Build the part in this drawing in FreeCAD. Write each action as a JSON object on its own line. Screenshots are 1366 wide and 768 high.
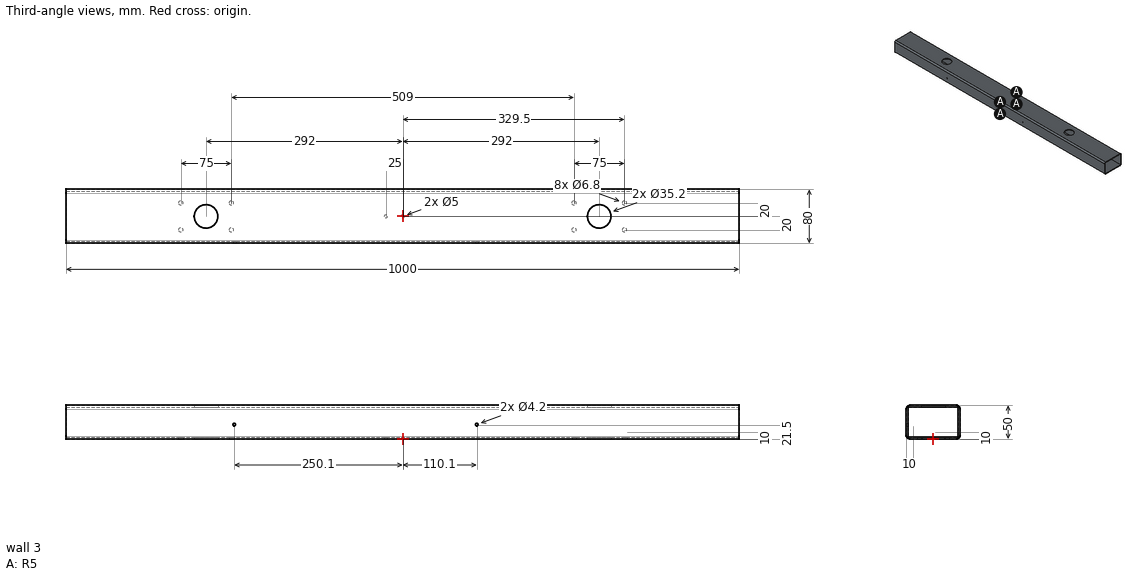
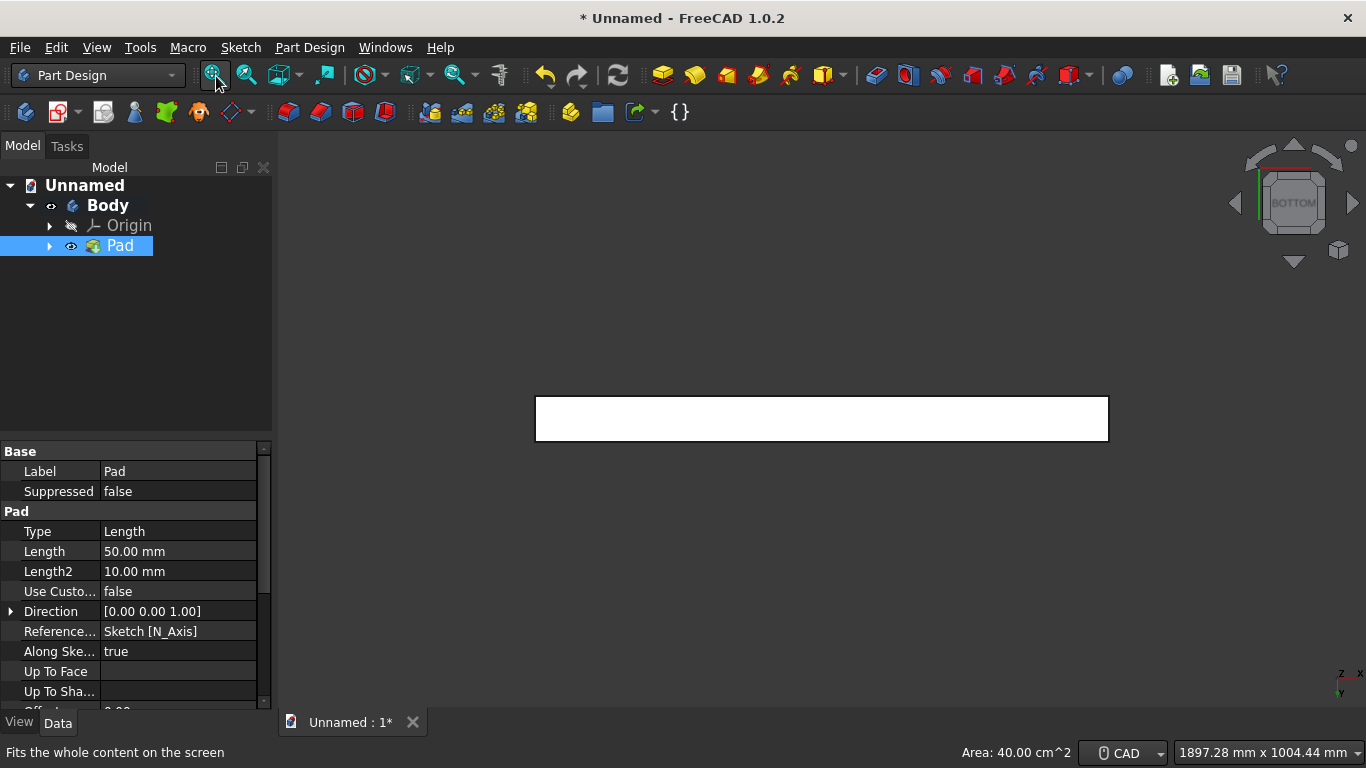
{"action": "key", "text": "4"}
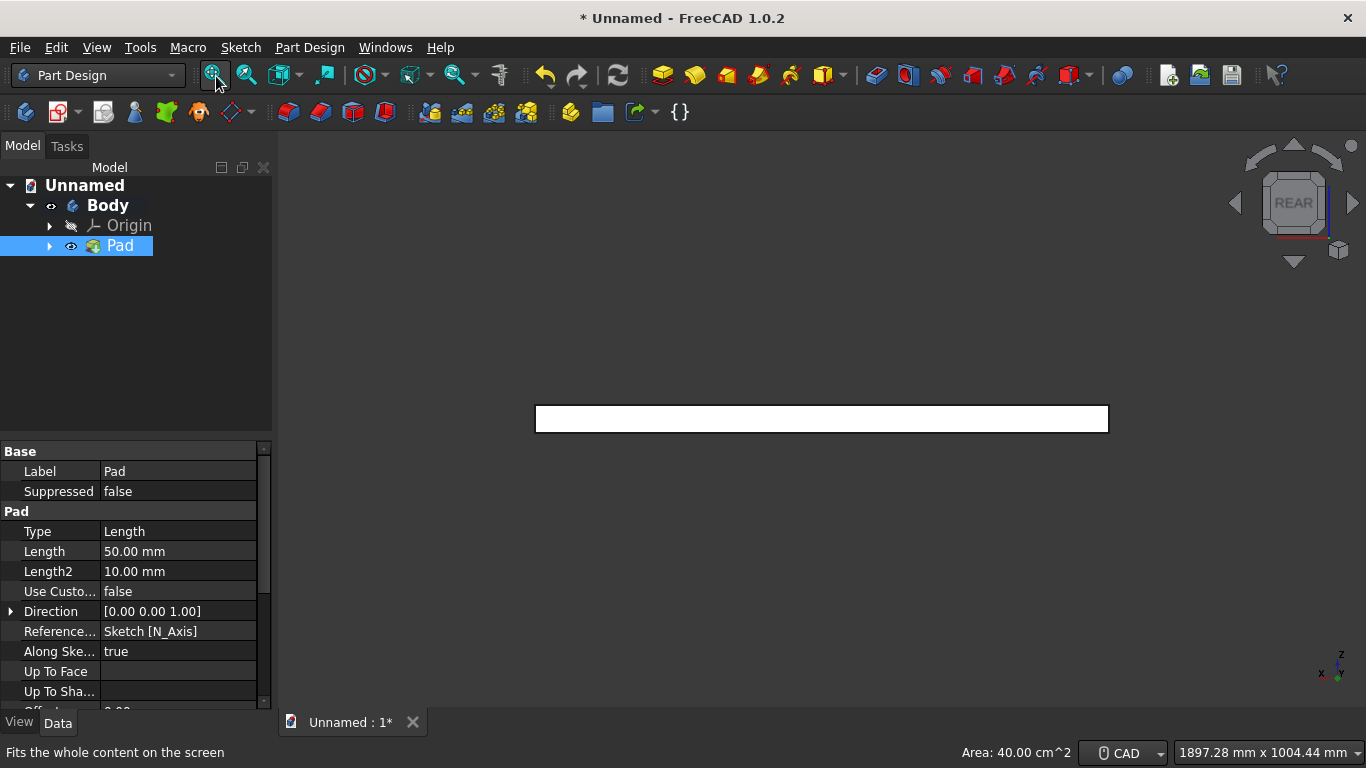
{"action": "key", "text": "6"}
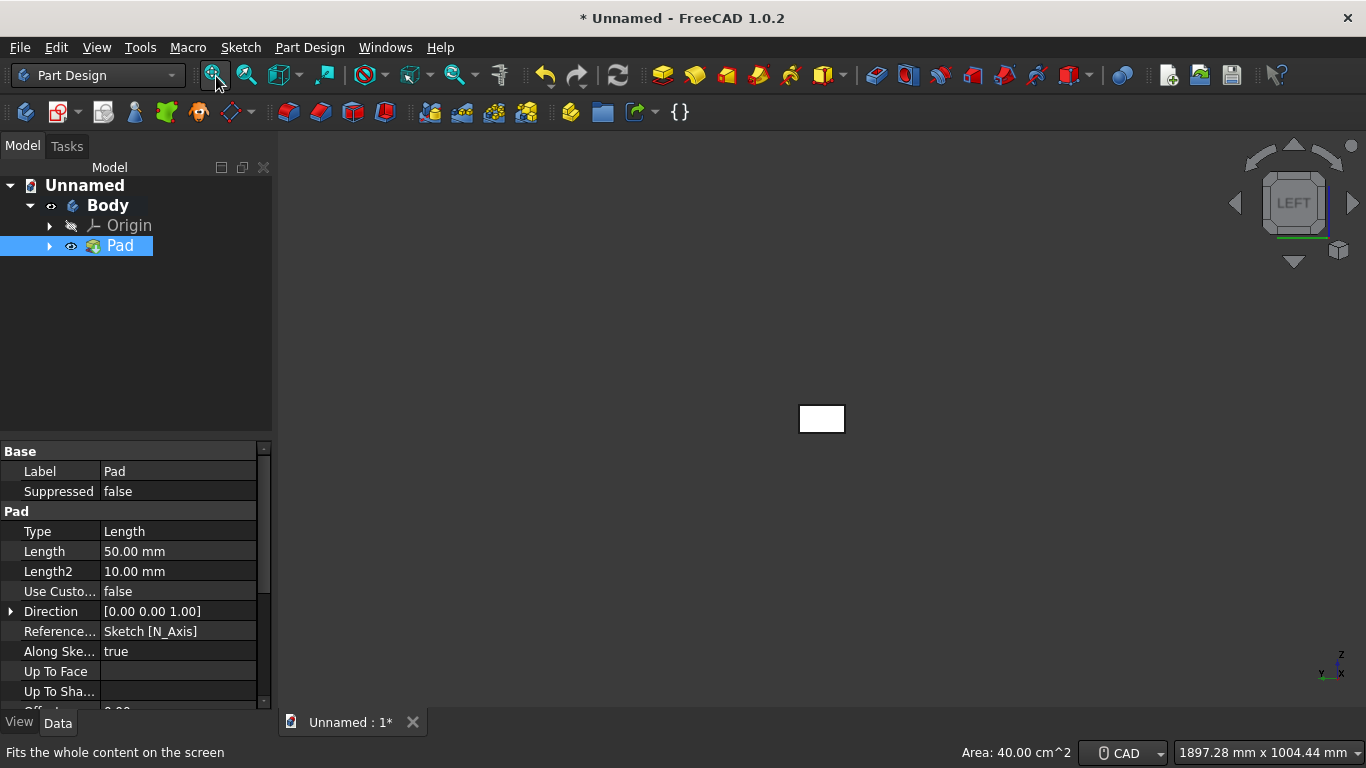
{"action": "left_click", "coordinate": [216, 76]}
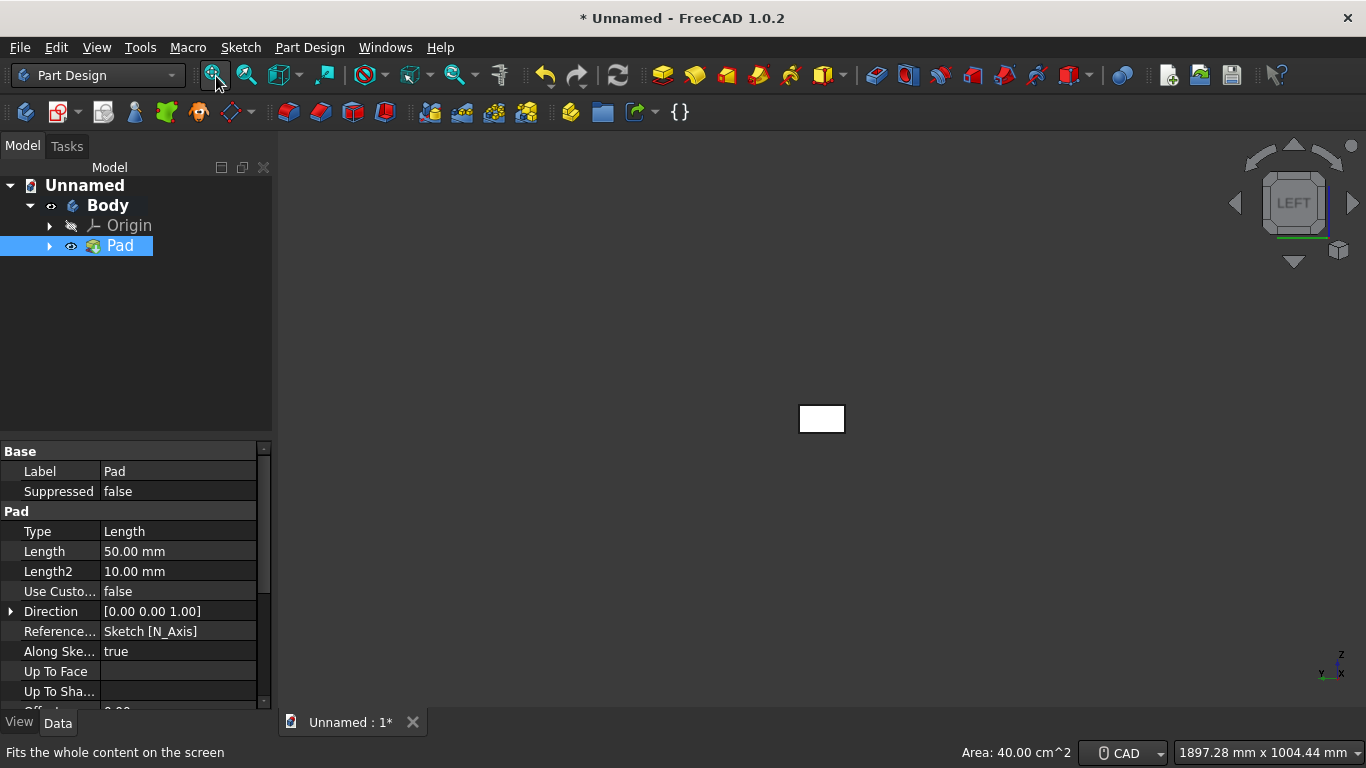
{"action": "left_click", "coordinate": [815, 418], "text": "ctrl"}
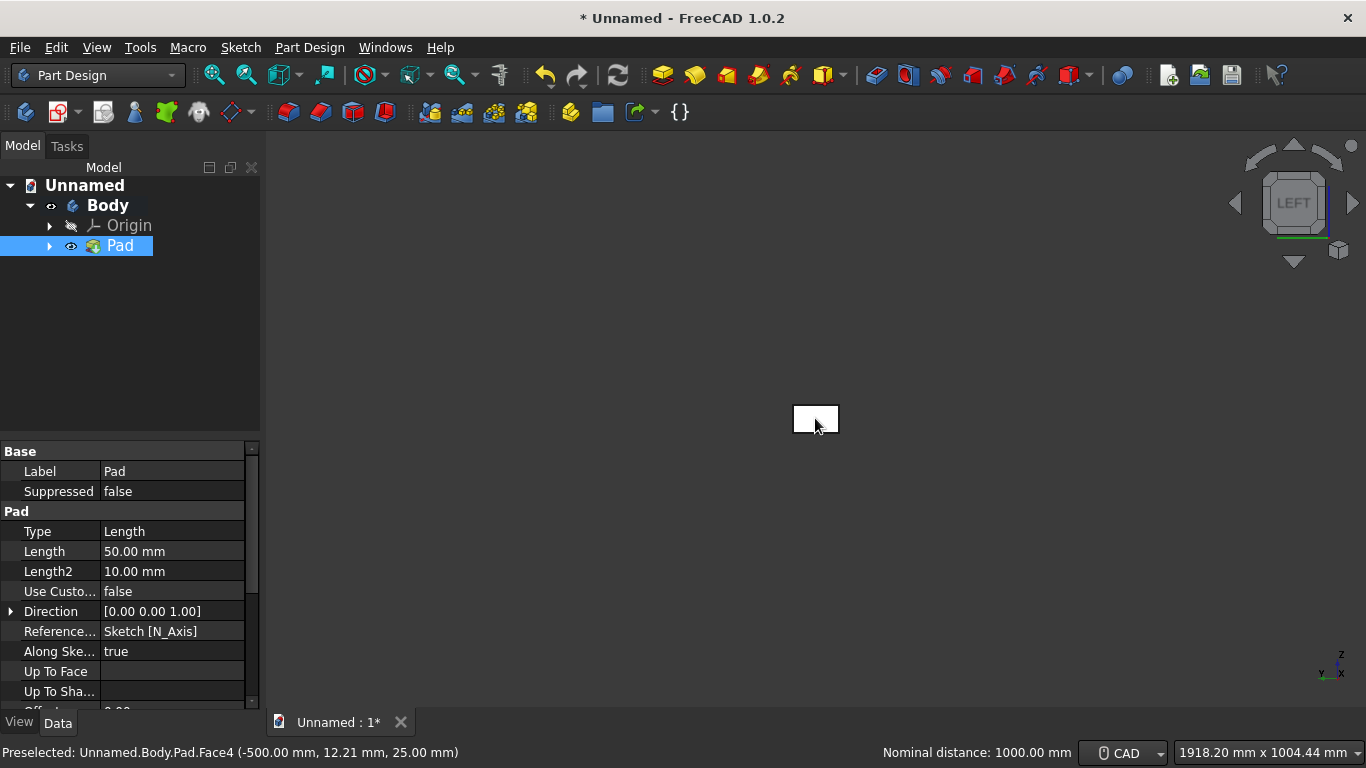
{"action": "left_click", "coordinate": [386, 112]}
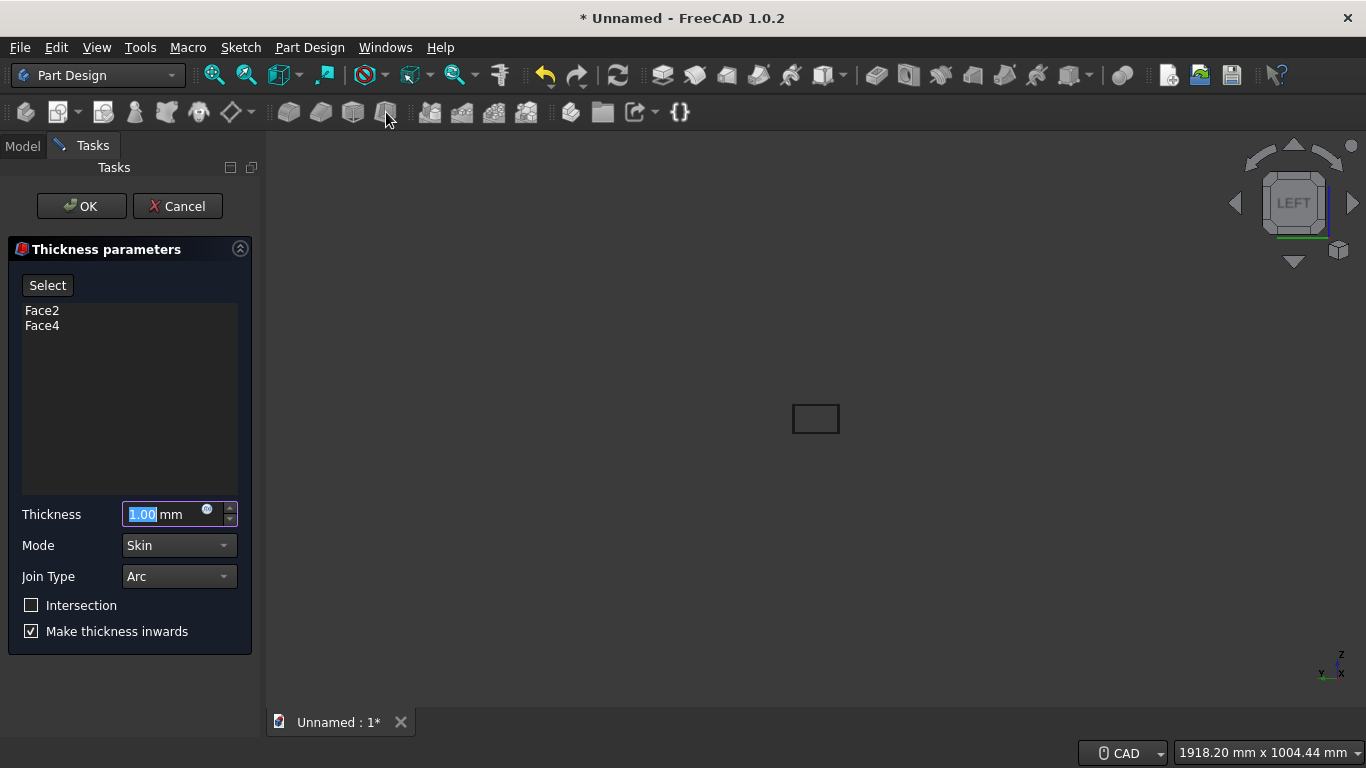
{"action": "type", "text": "3"}
{"action": "key", "text": "Tab"}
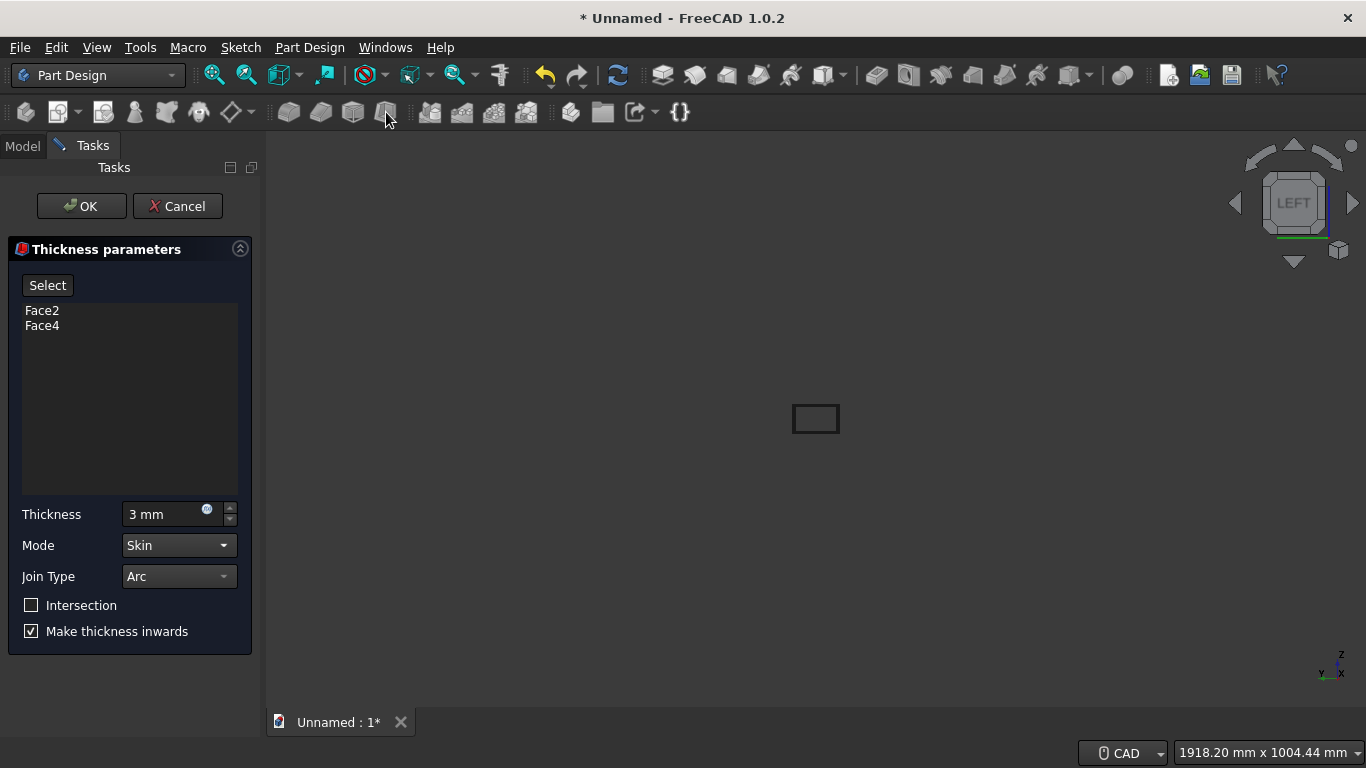
{"action": "left_click", "coordinate": [180, 576]}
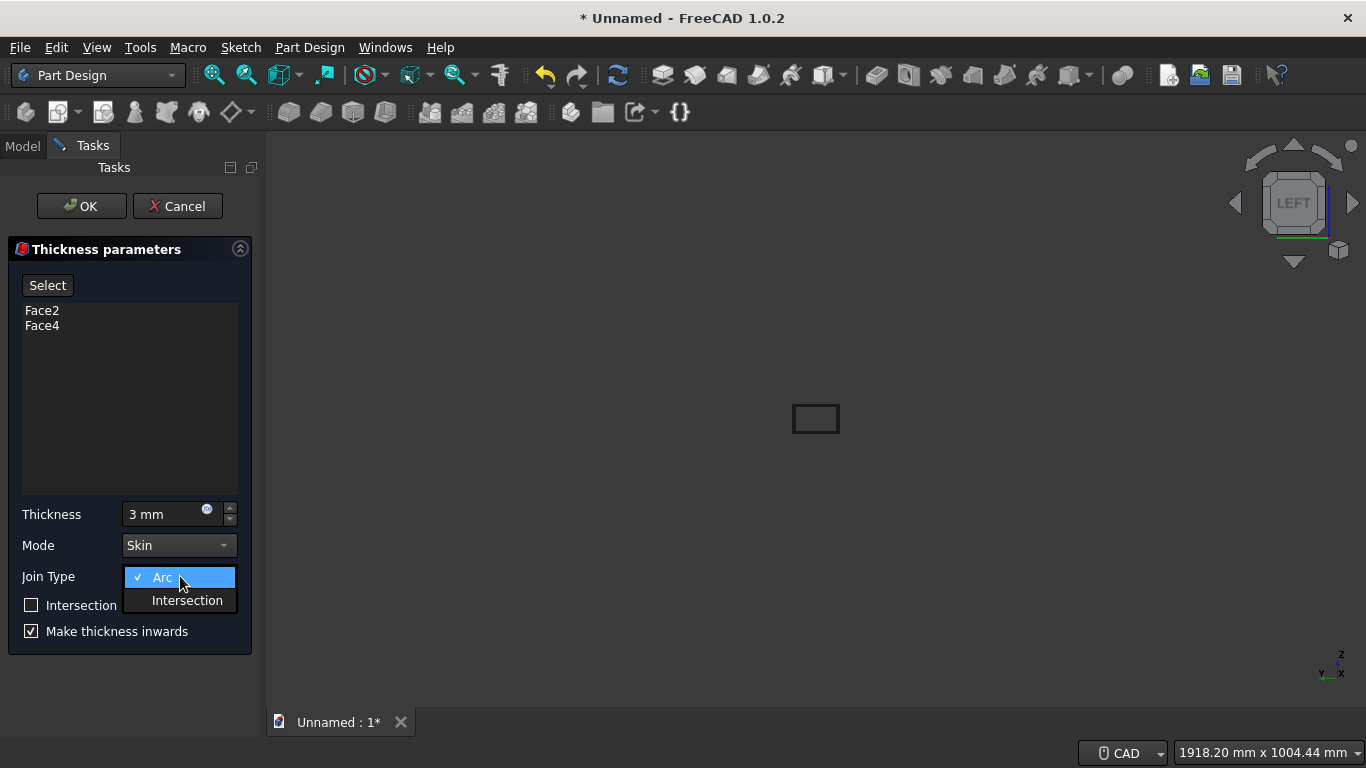
{"action": "left_click", "coordinate": [179, 600]}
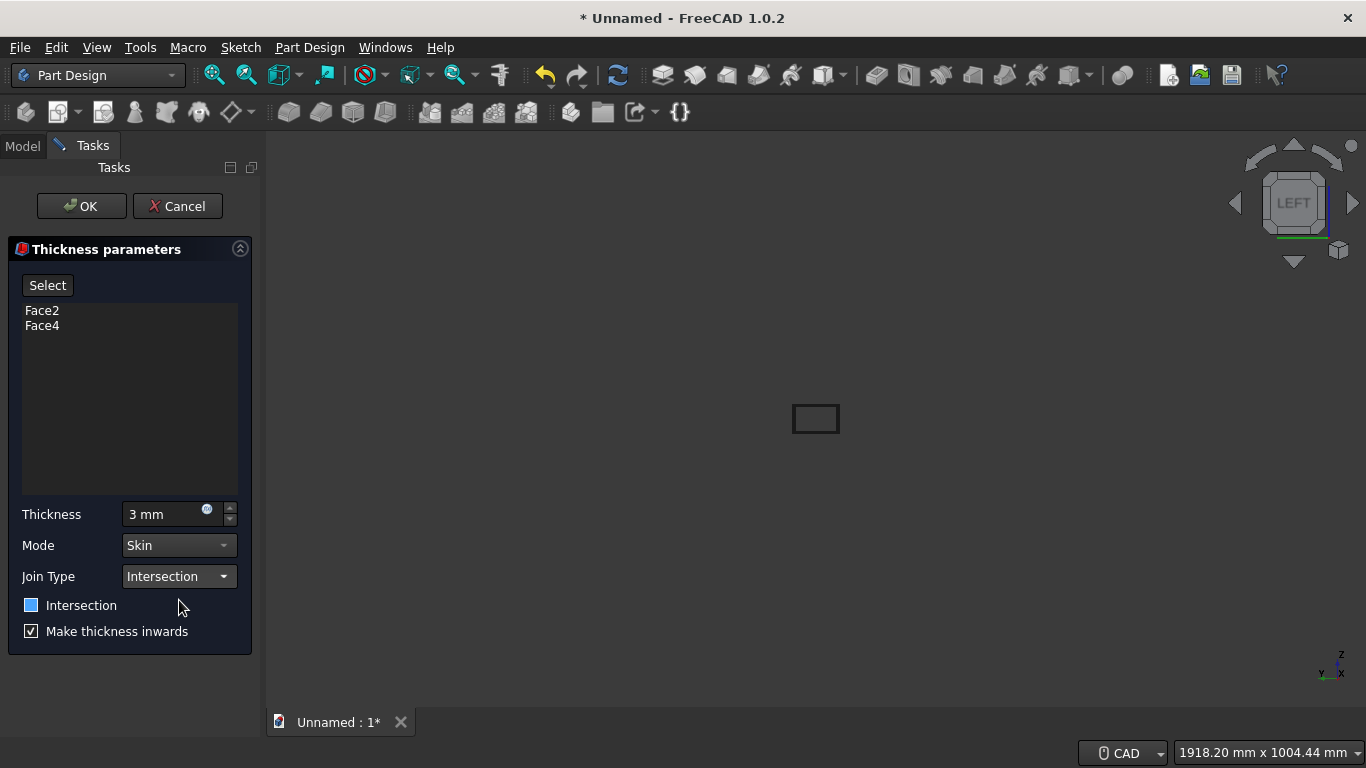
{"action": "left_click", "coordinate": [82, 206]}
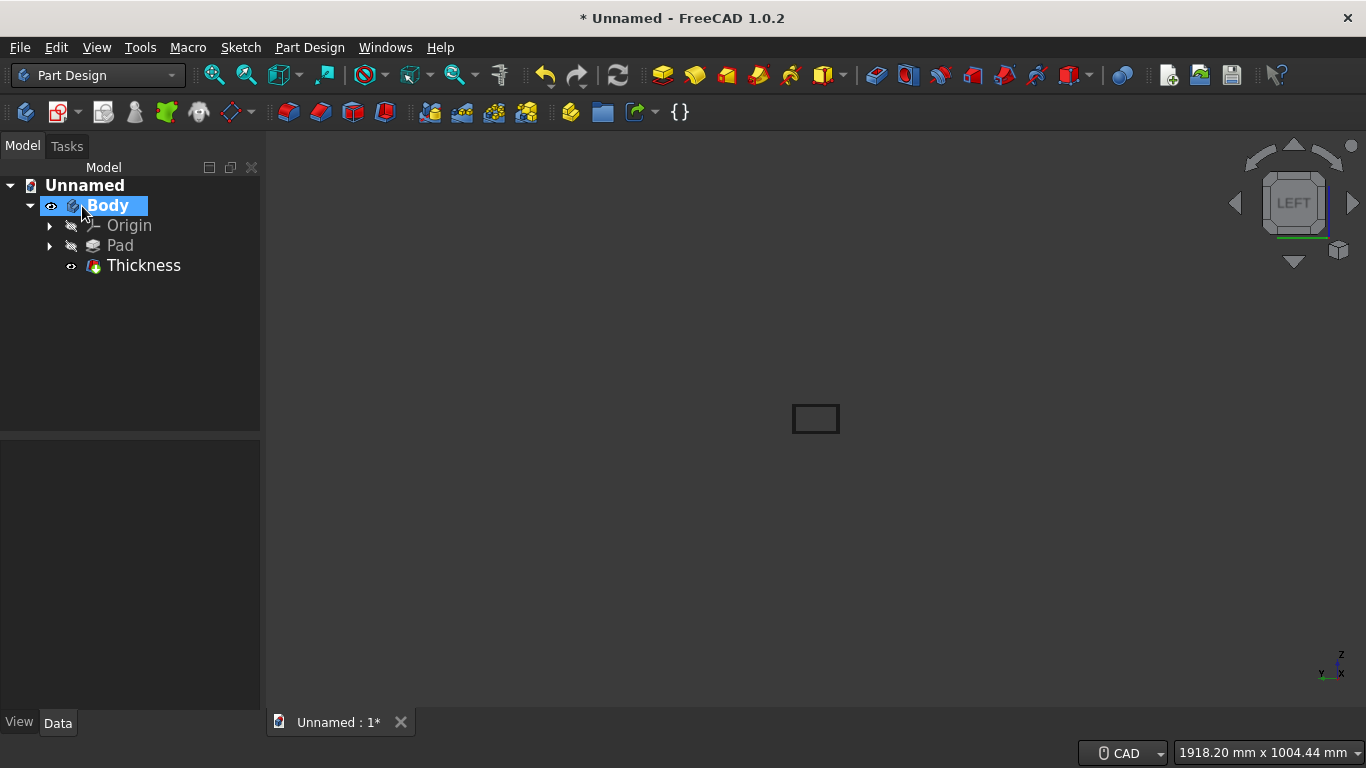
{"action": "left_click", "coordinate": [216, 76]}